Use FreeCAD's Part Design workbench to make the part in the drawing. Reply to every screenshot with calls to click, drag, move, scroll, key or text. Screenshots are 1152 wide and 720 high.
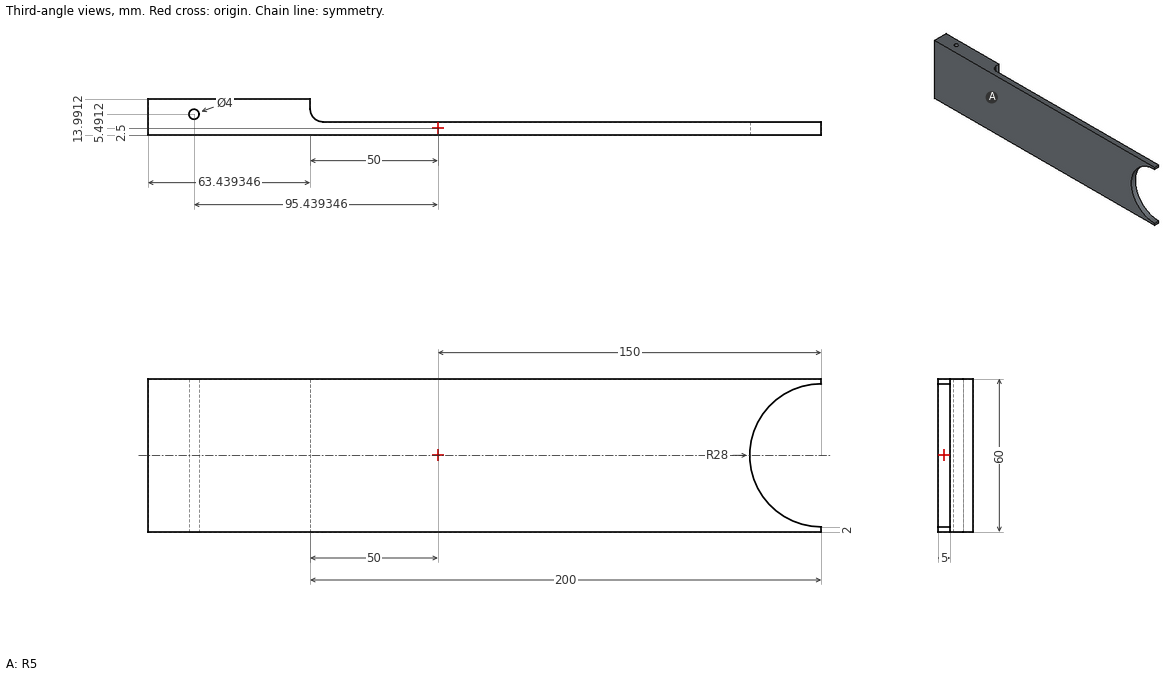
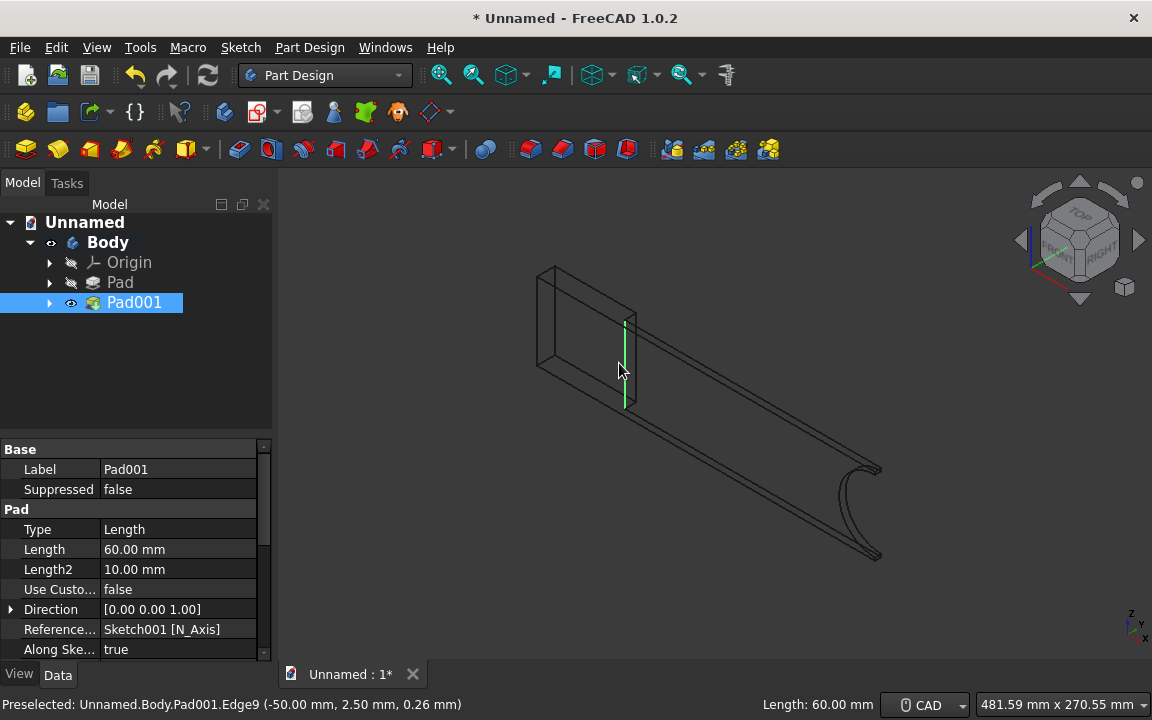
key(v)
key(1)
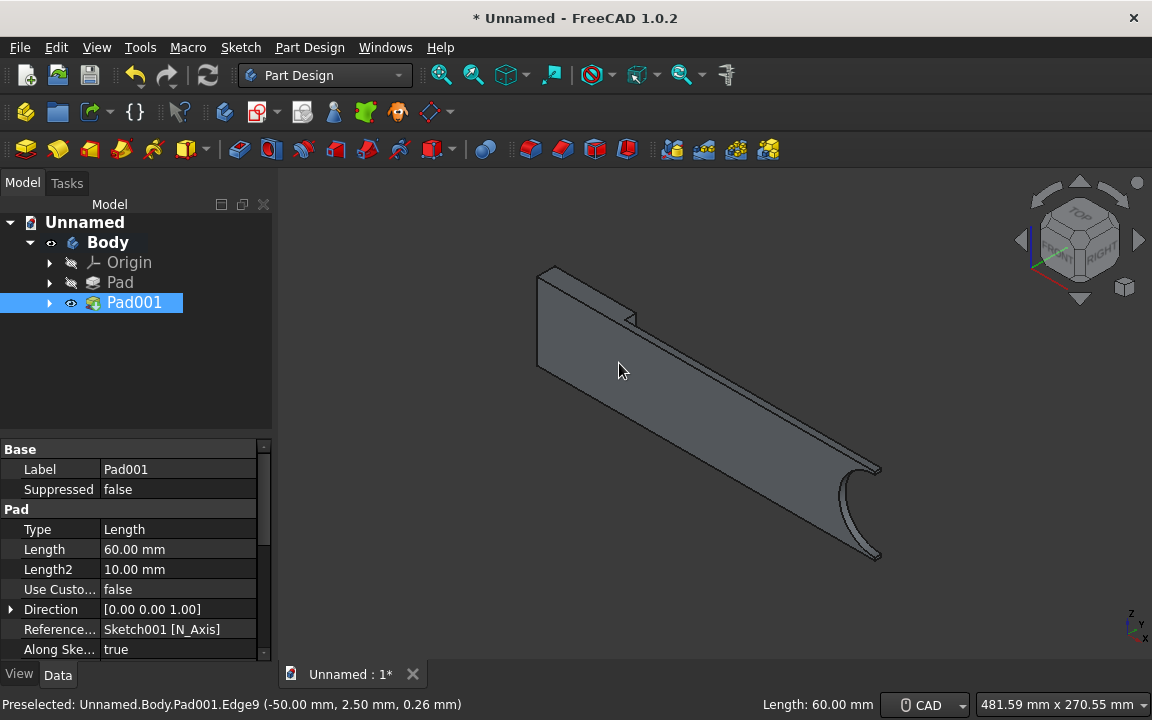
click(532, 150)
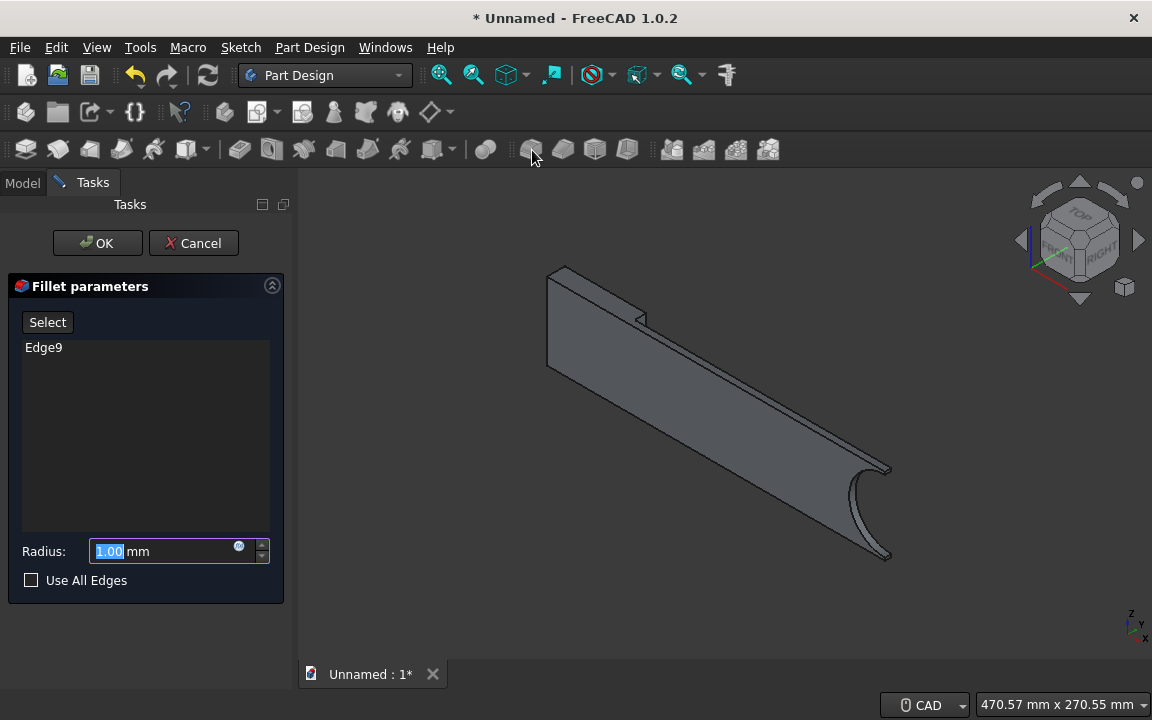
text(5)
key(Tab)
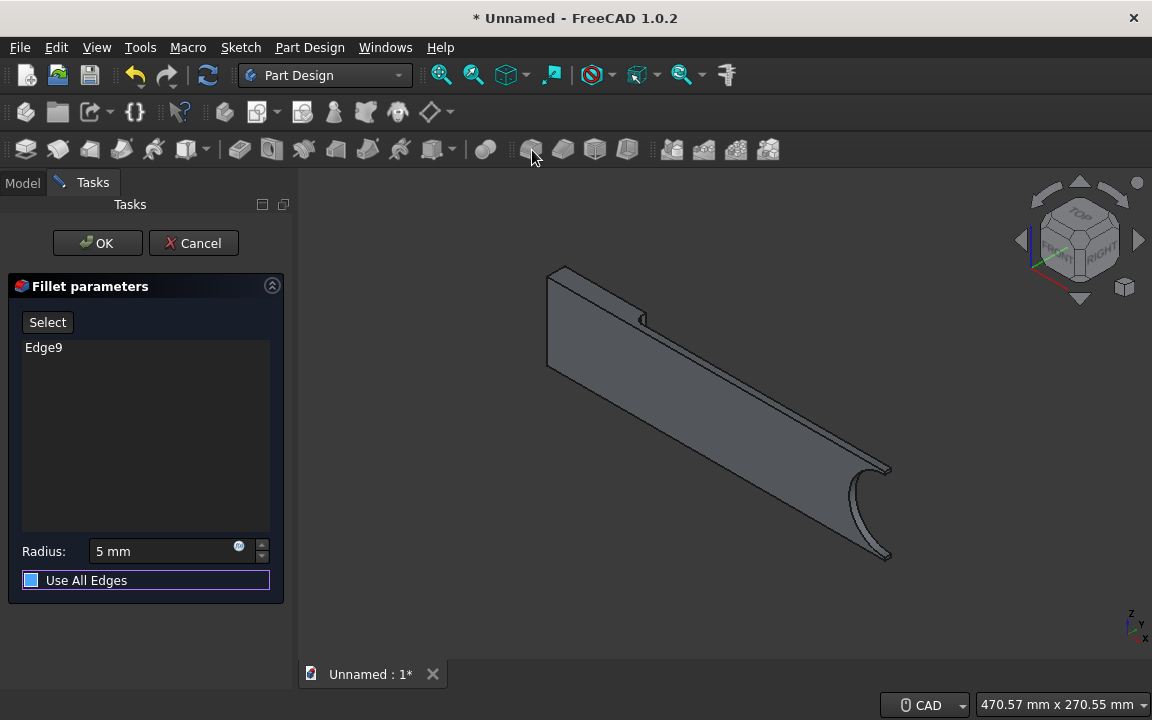
click(98, 243)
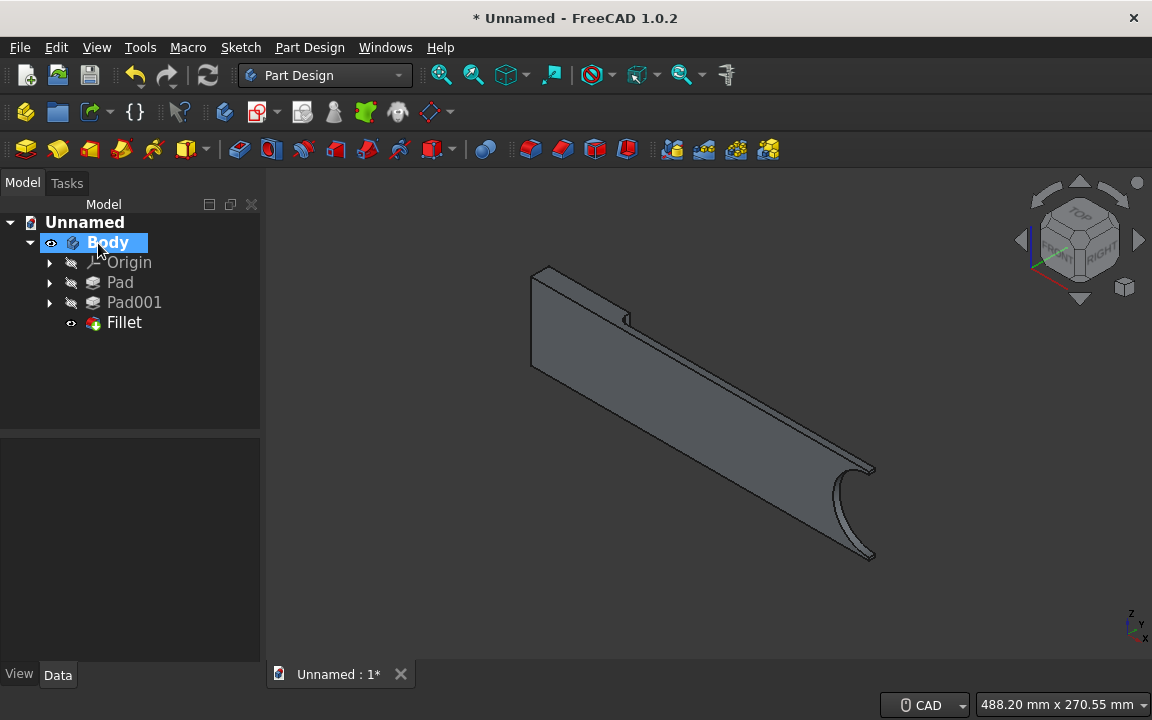
click(564, 284)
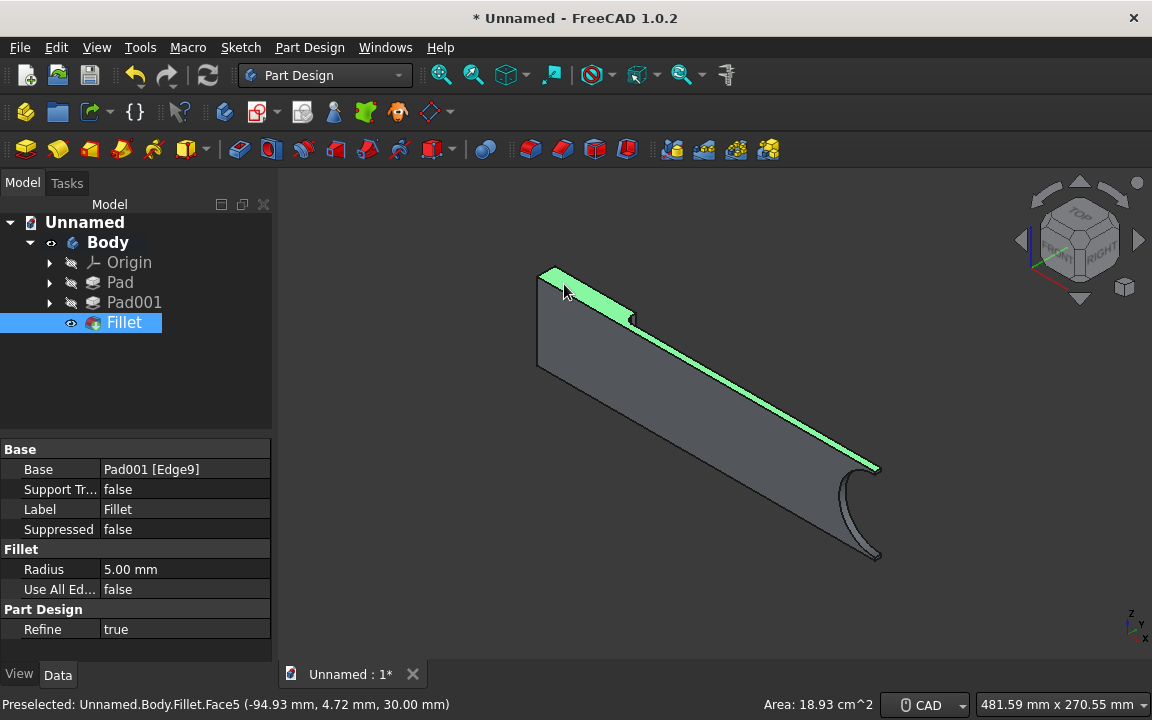
click(258, 112)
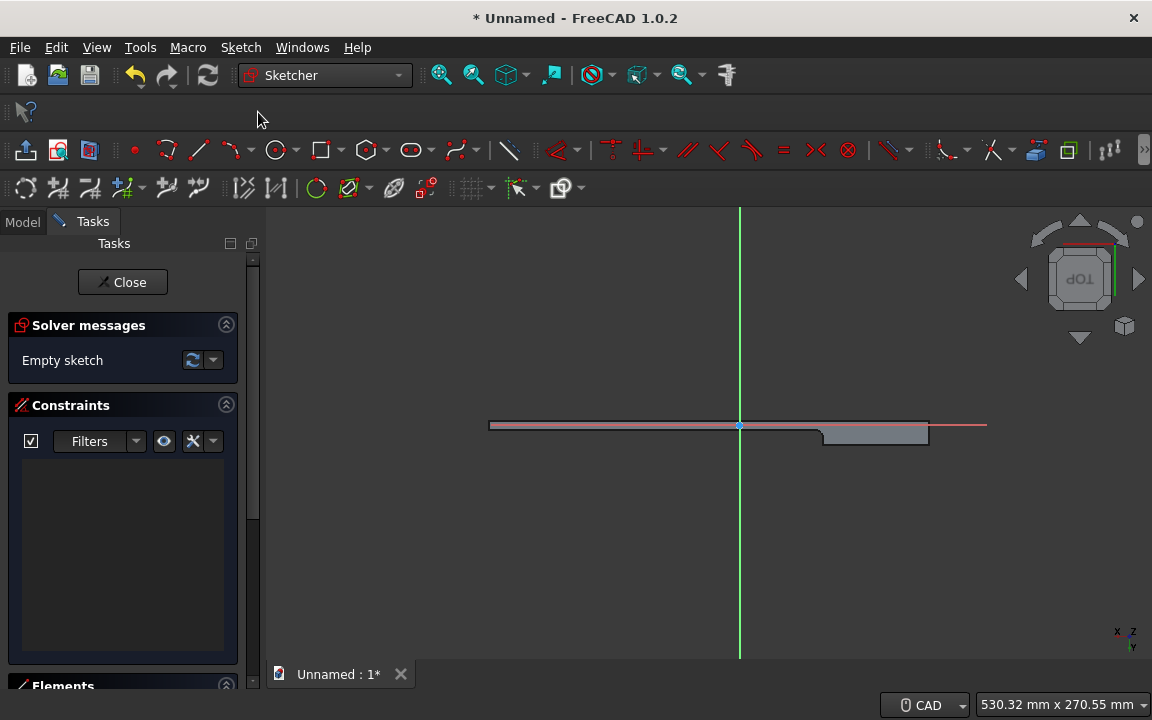
scroll(913, 435, up, 15)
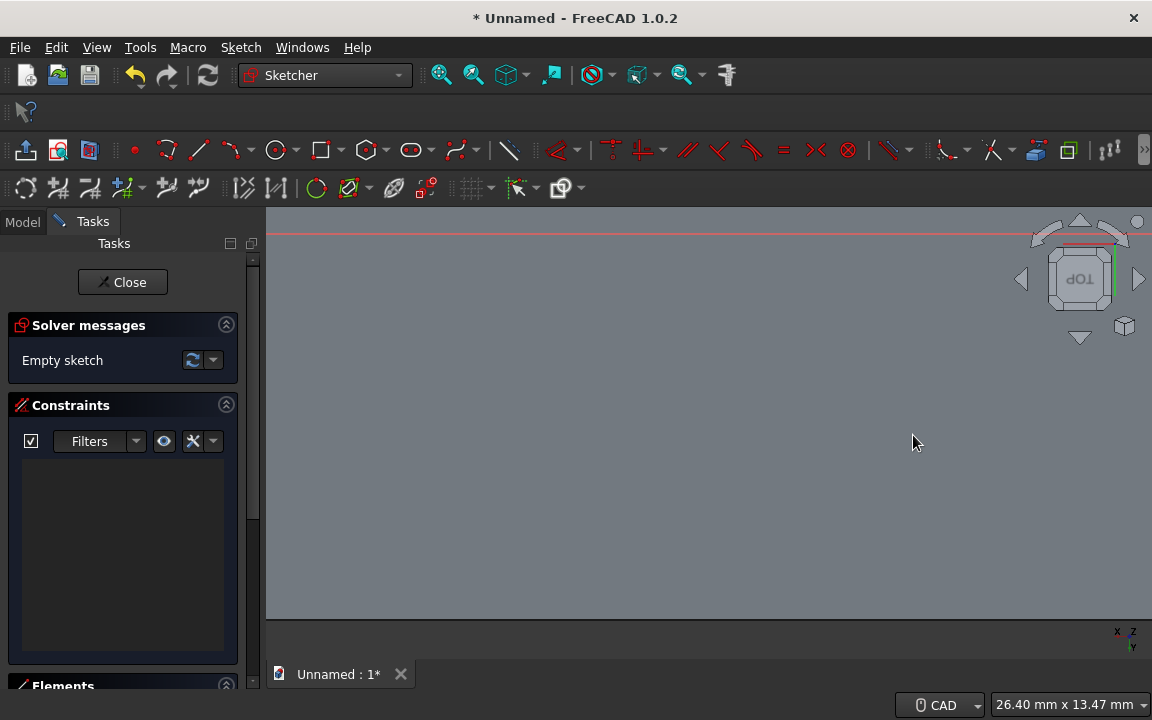
scroll(599, 407, up, 4)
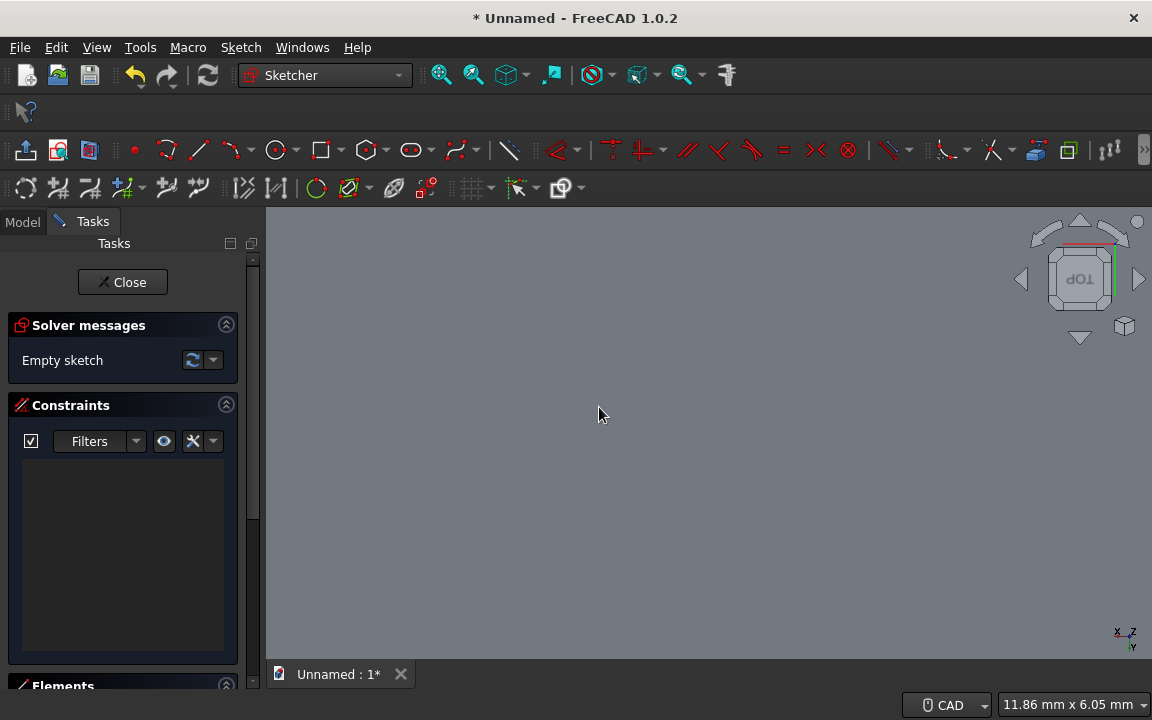
key(g)
key(c)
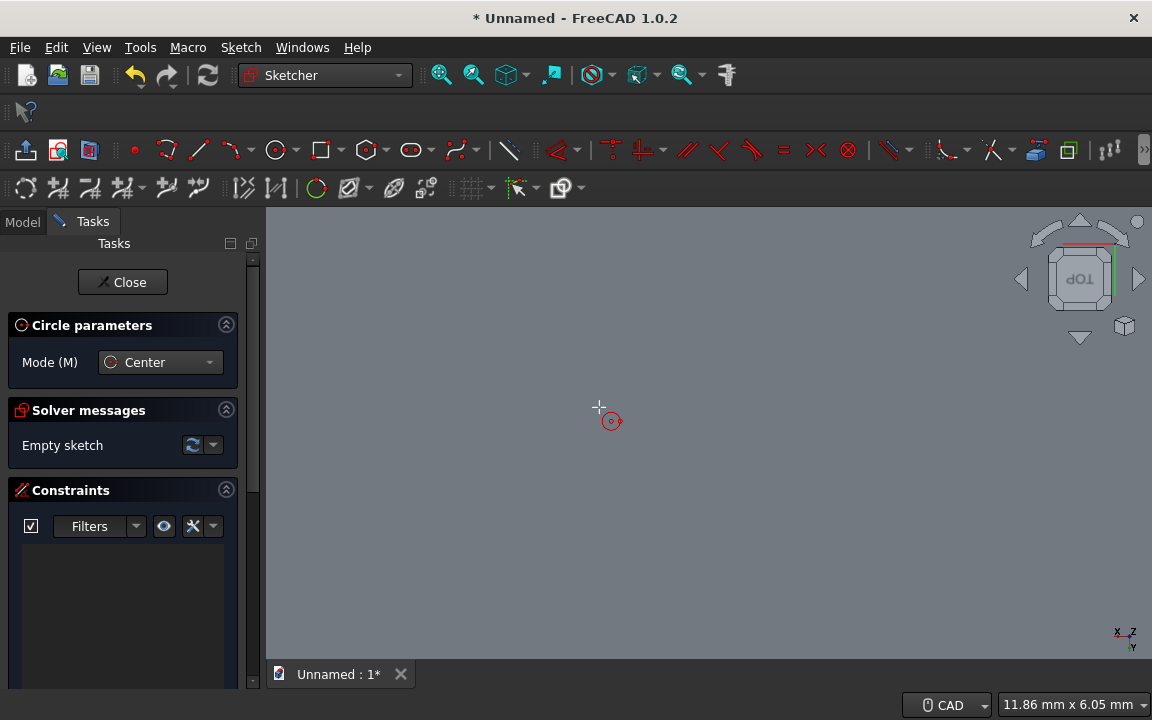
click(640, 432)
move(746, 327)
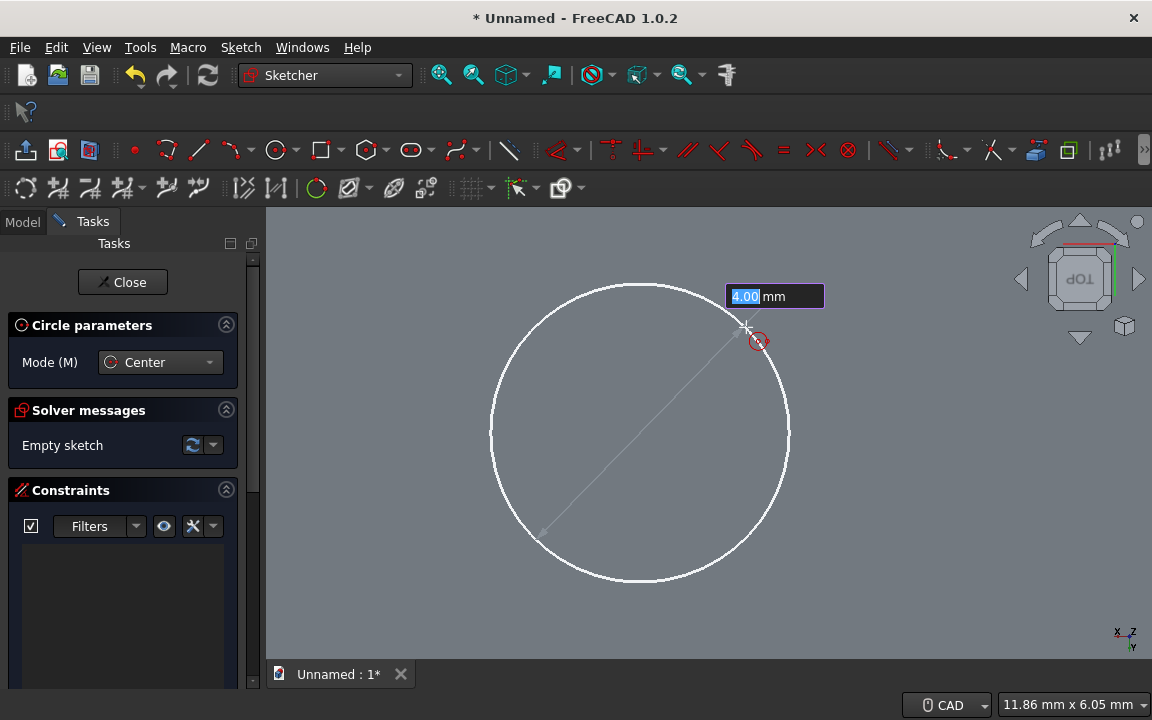
text(4)
key(Return)
key(Escape)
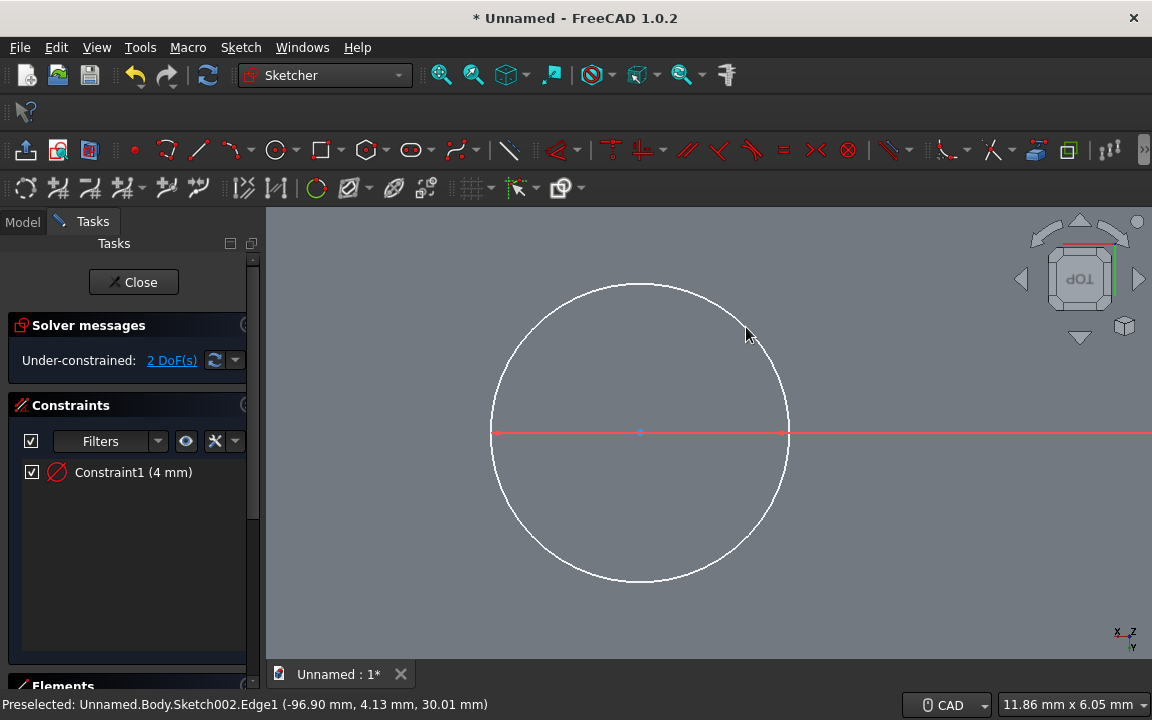
click(556, 150)